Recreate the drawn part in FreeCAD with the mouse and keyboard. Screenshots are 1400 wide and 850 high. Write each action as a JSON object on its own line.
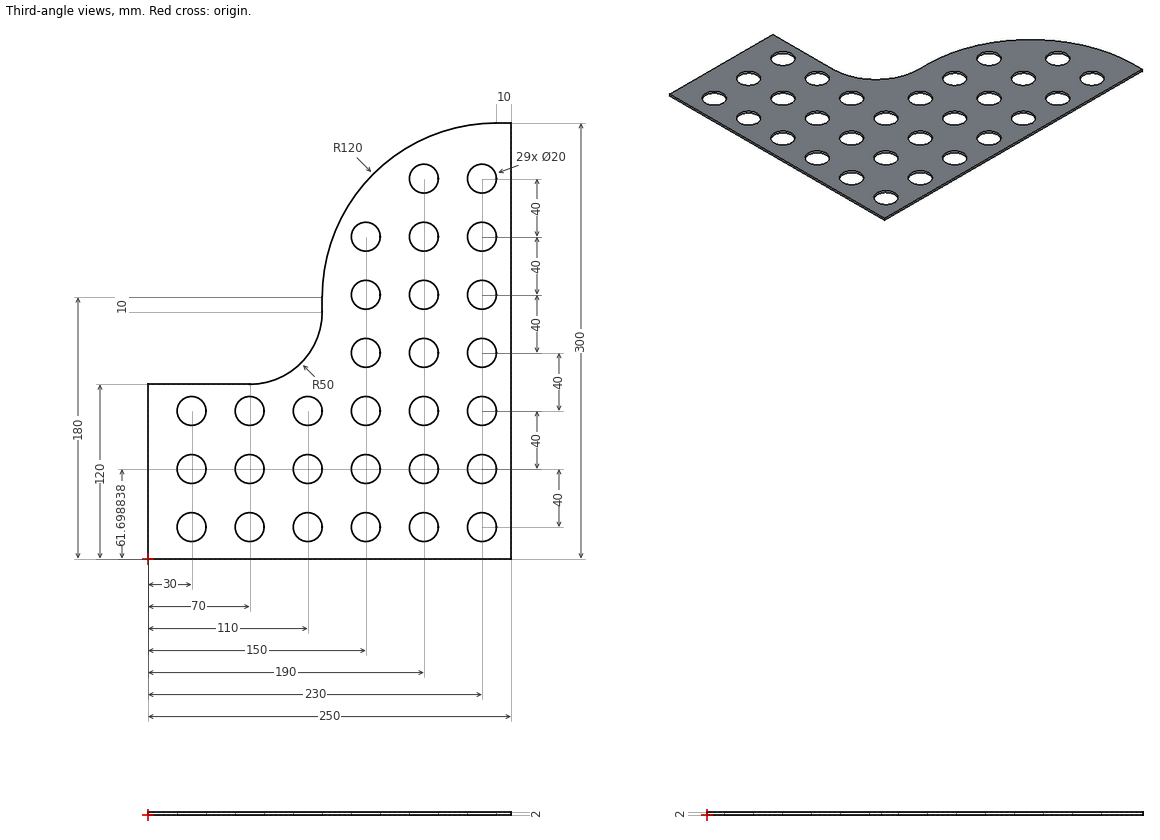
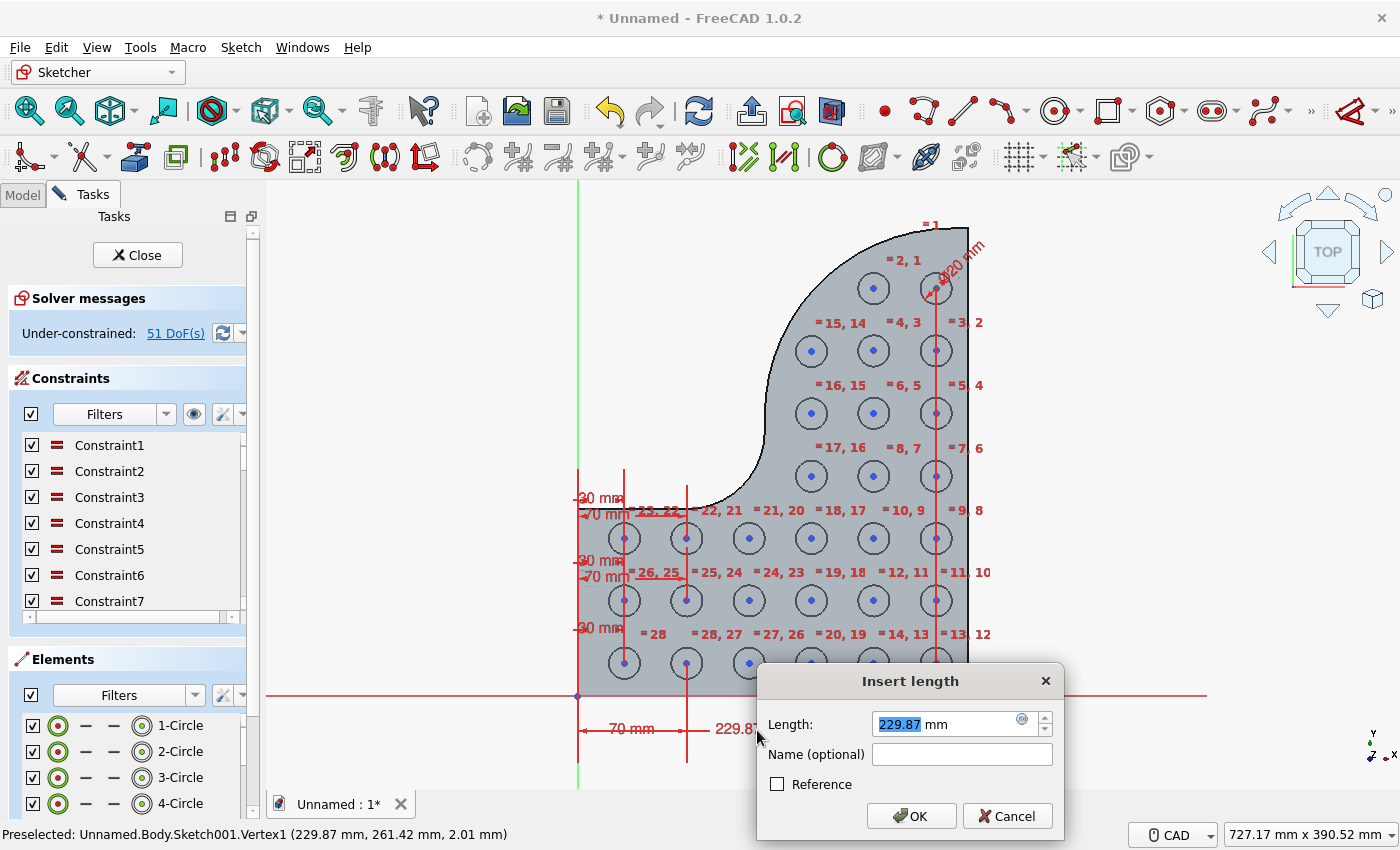
{"action": "type", "text": "230"}
{"action": "key", "text": "Return"}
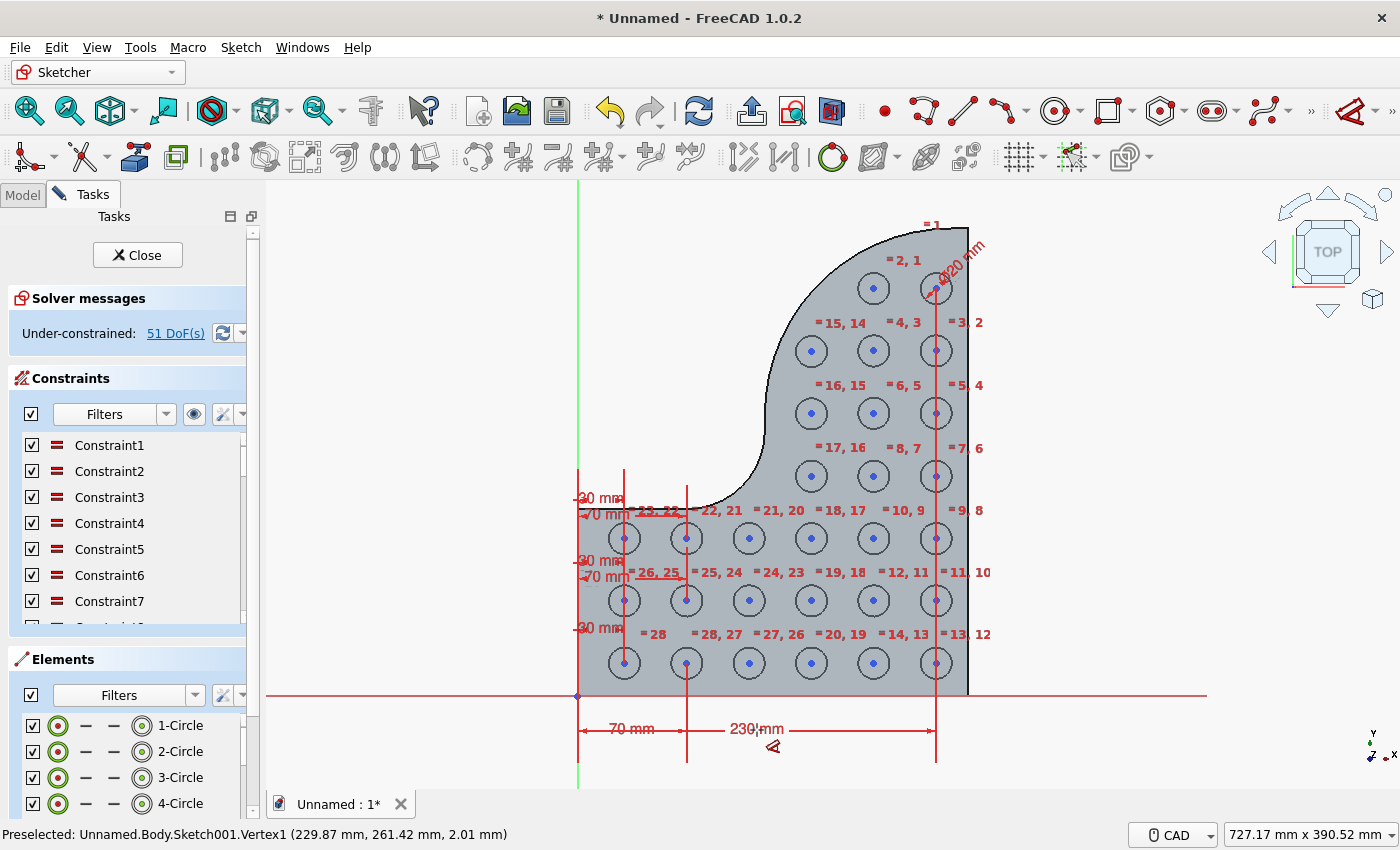
{"action": "left_click", "coordinate": [874, 289]}
{"action": "left_click", "coordinate": [829, 730]}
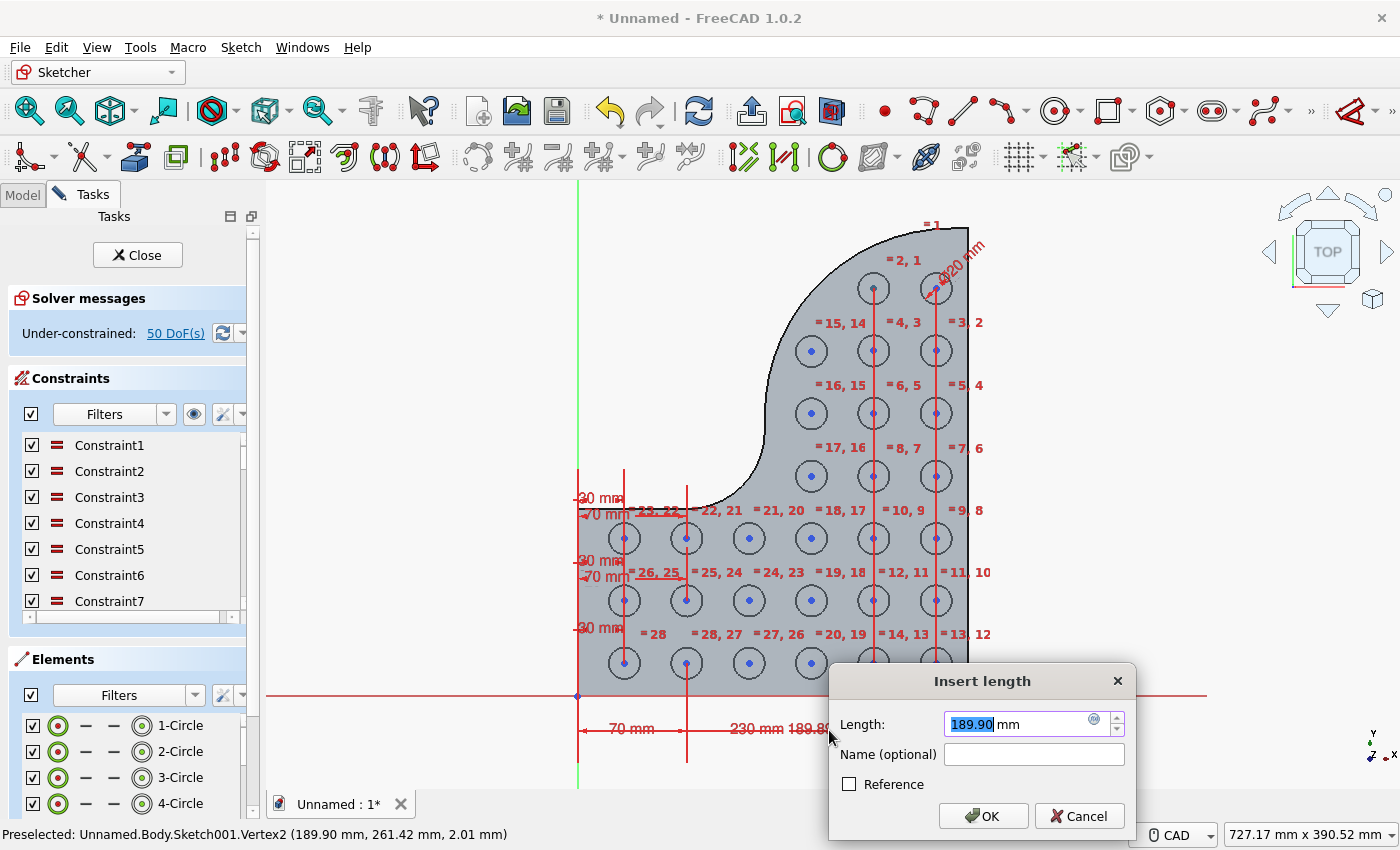
{"action": "type", "text": "190"}
{"action": "key", "text": "Return"}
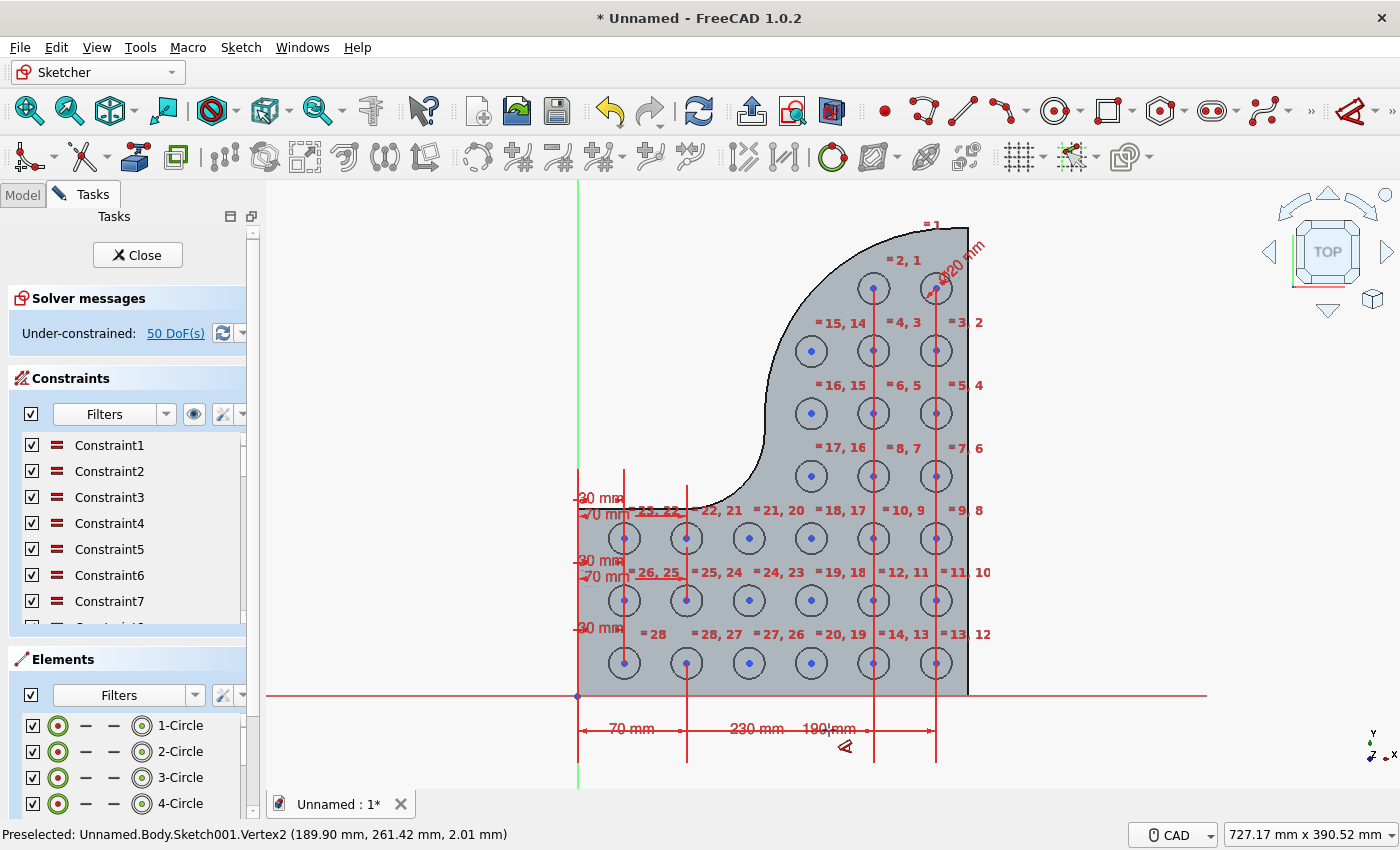
{"action": "left_click", "coordinate": [936, 351]}
{"action": "left_click", "coordinate": [757, 317]}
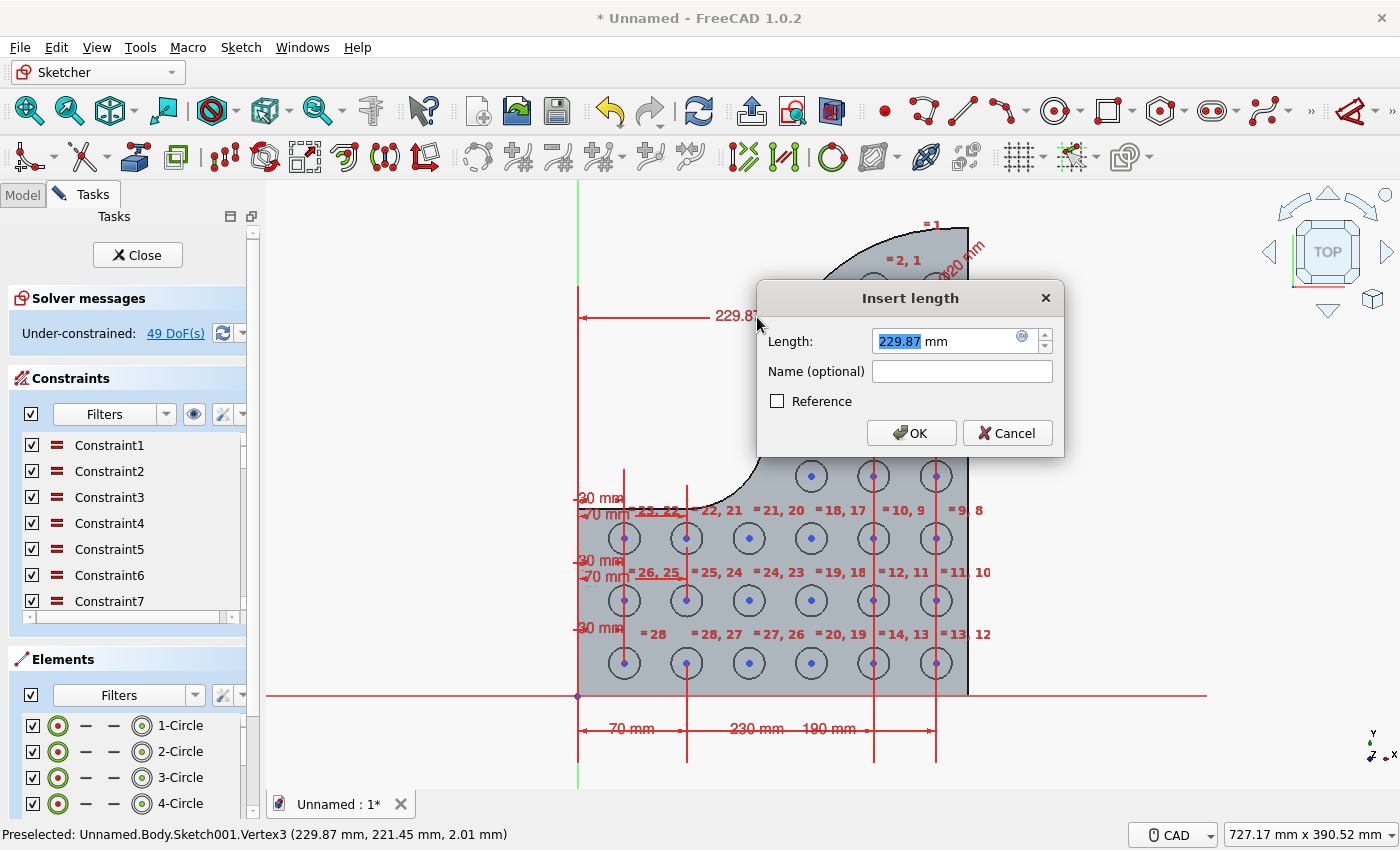
{"action": "type", "text": "230"}
{"action": "key", "text": "Return"}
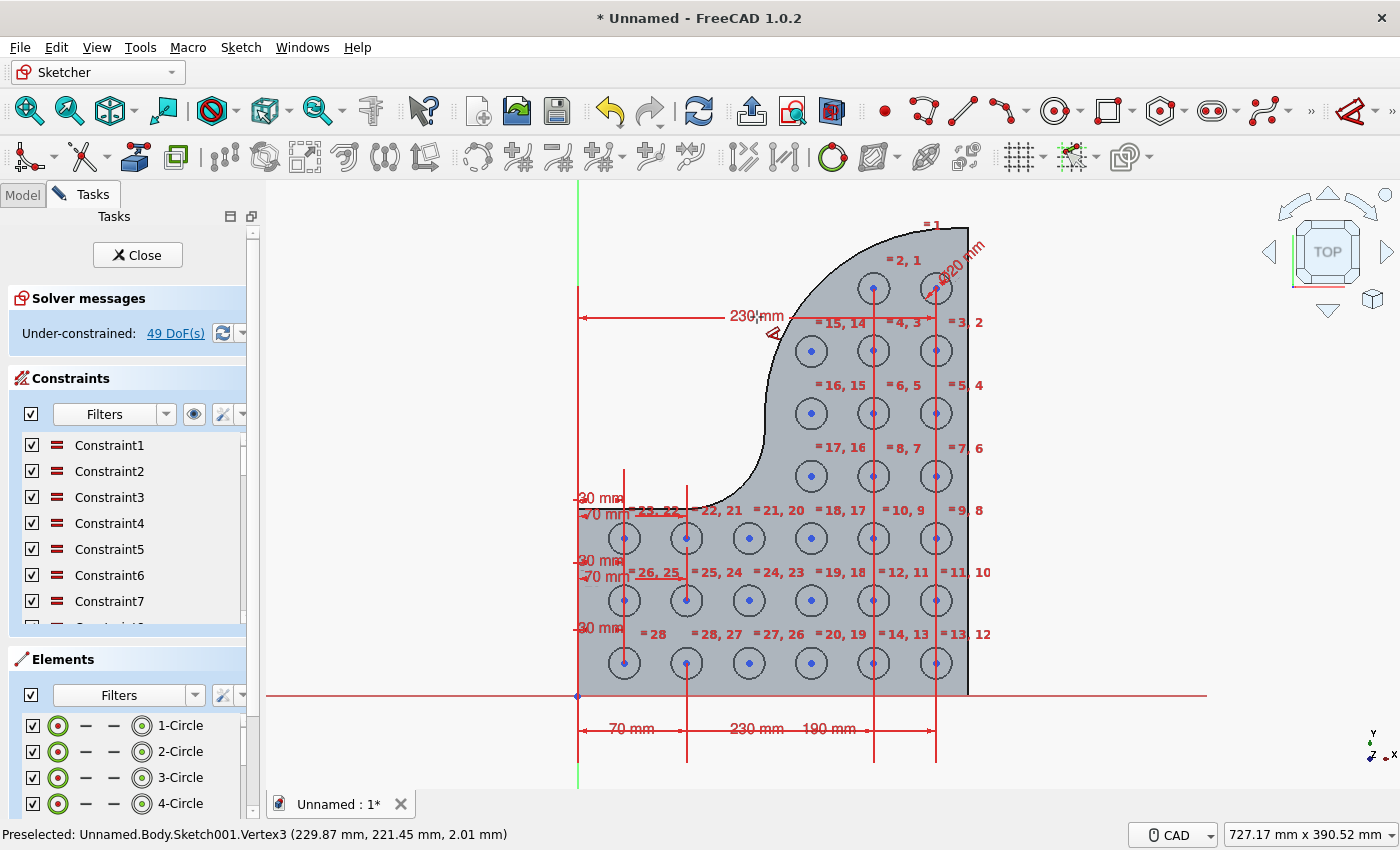
{"action": "left_click", "coordinate": [874, 351]}
{"action": "left_click", "coordinate": [658, 317]}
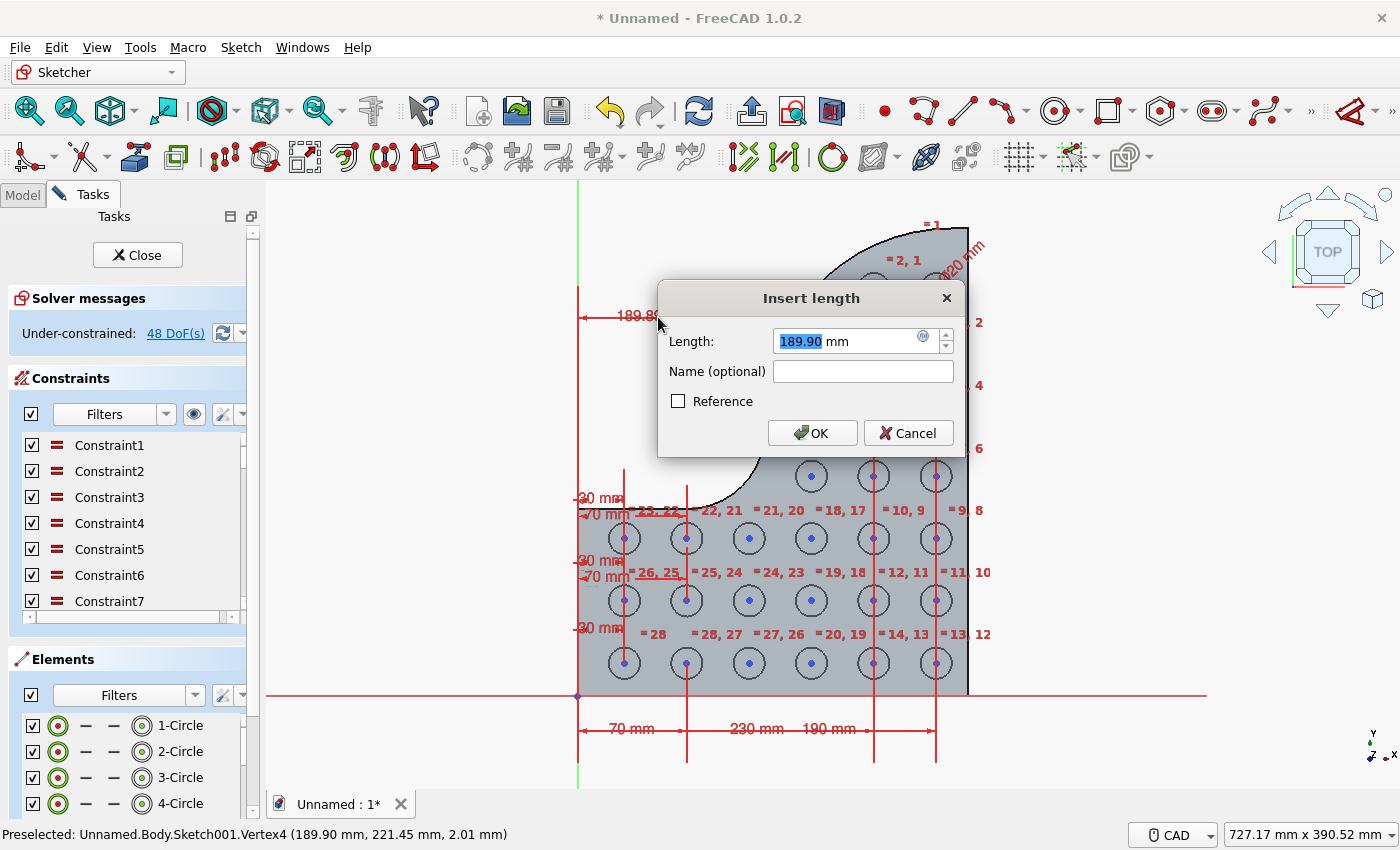
{"action": "type", "text": "190"}
{"action": "key", "text": "Return"}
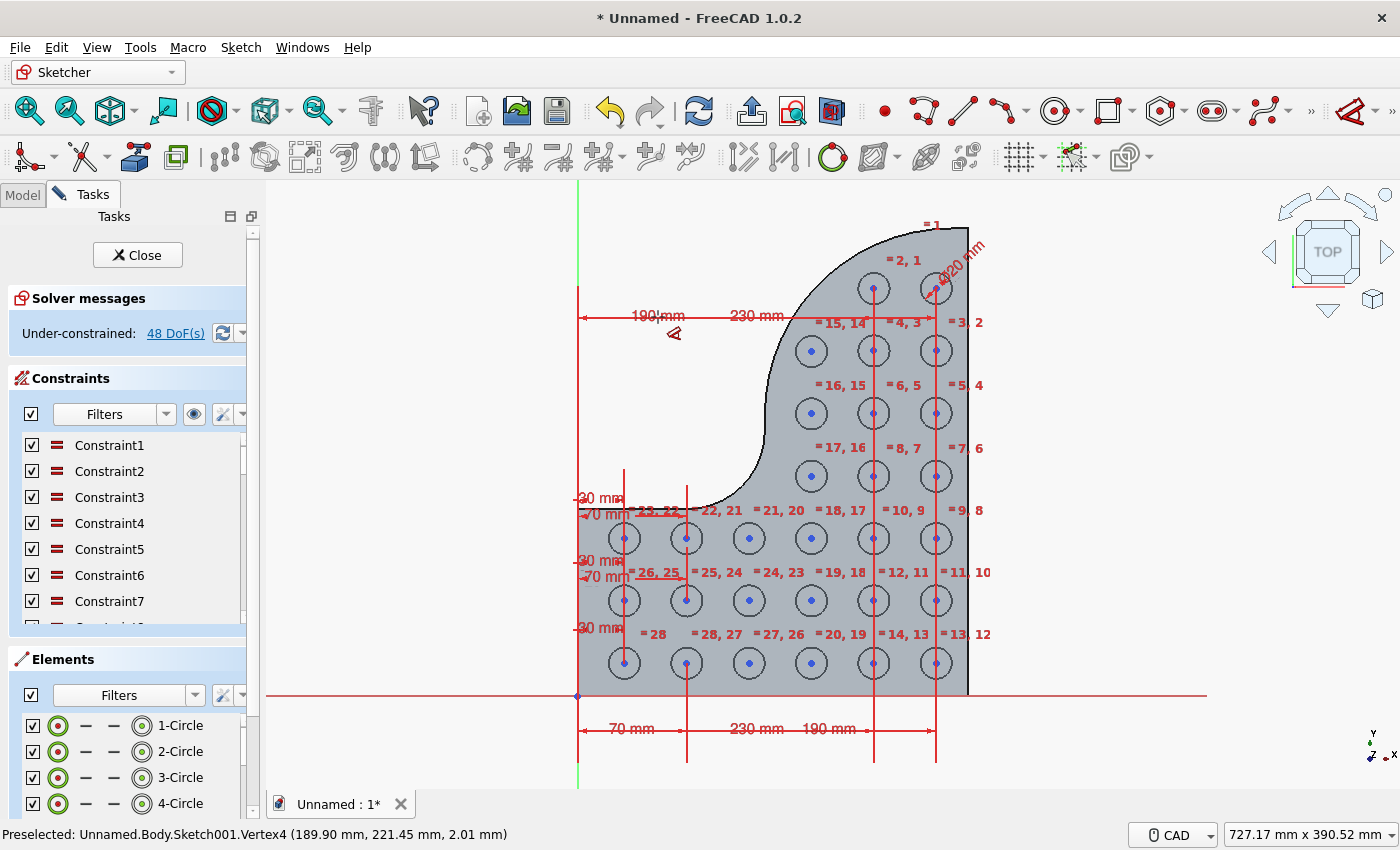
{"action": "left_click", "coordinate": [936, 413]}
{"action": "left_click", "coordinate": [757, 379]}